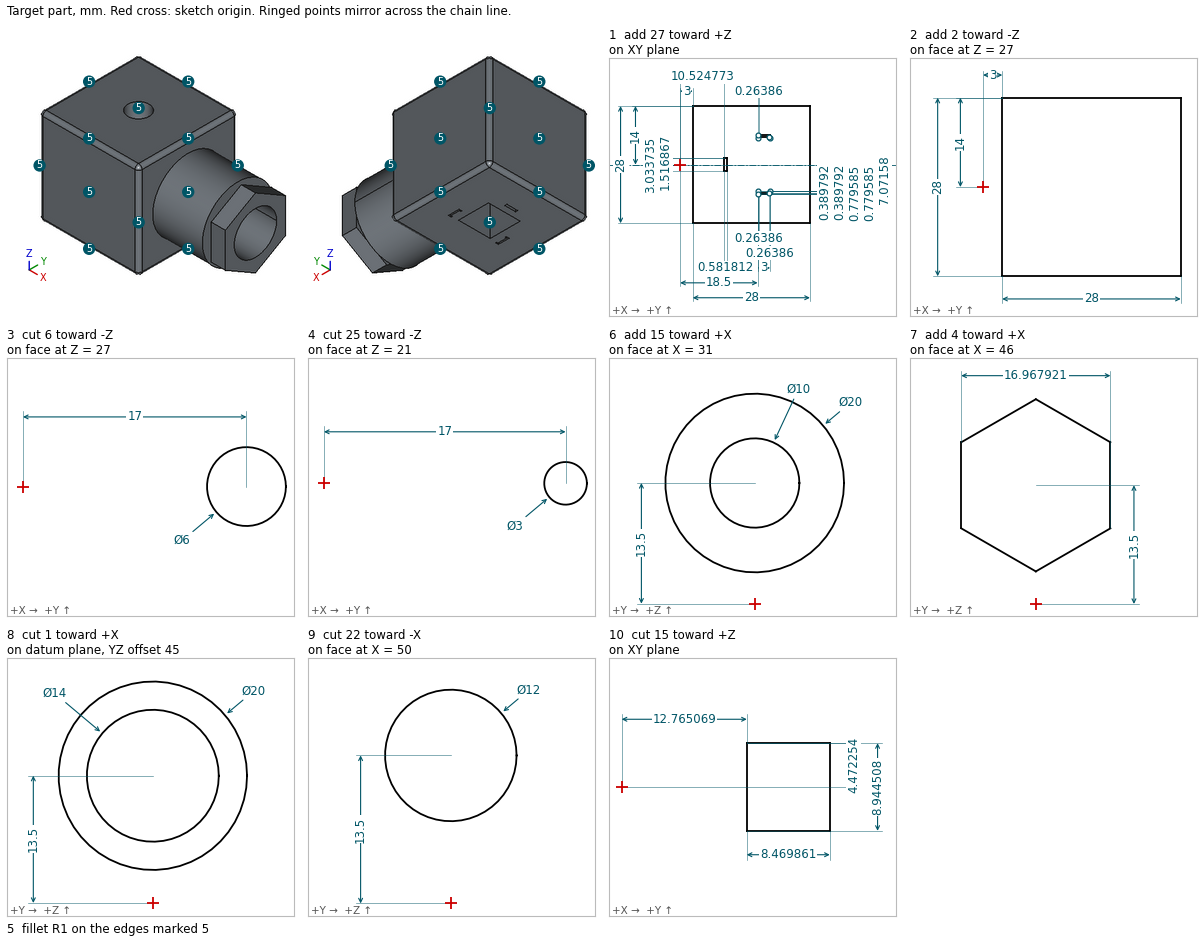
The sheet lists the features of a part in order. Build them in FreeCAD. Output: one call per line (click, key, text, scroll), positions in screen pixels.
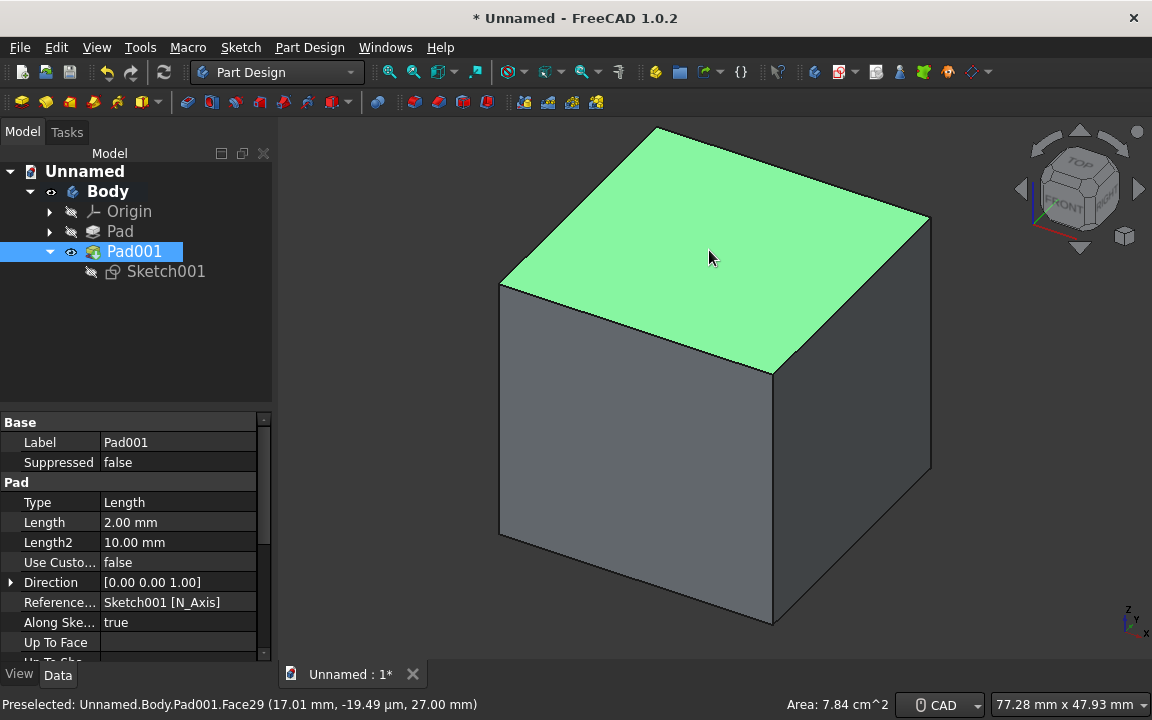
click(840, 72)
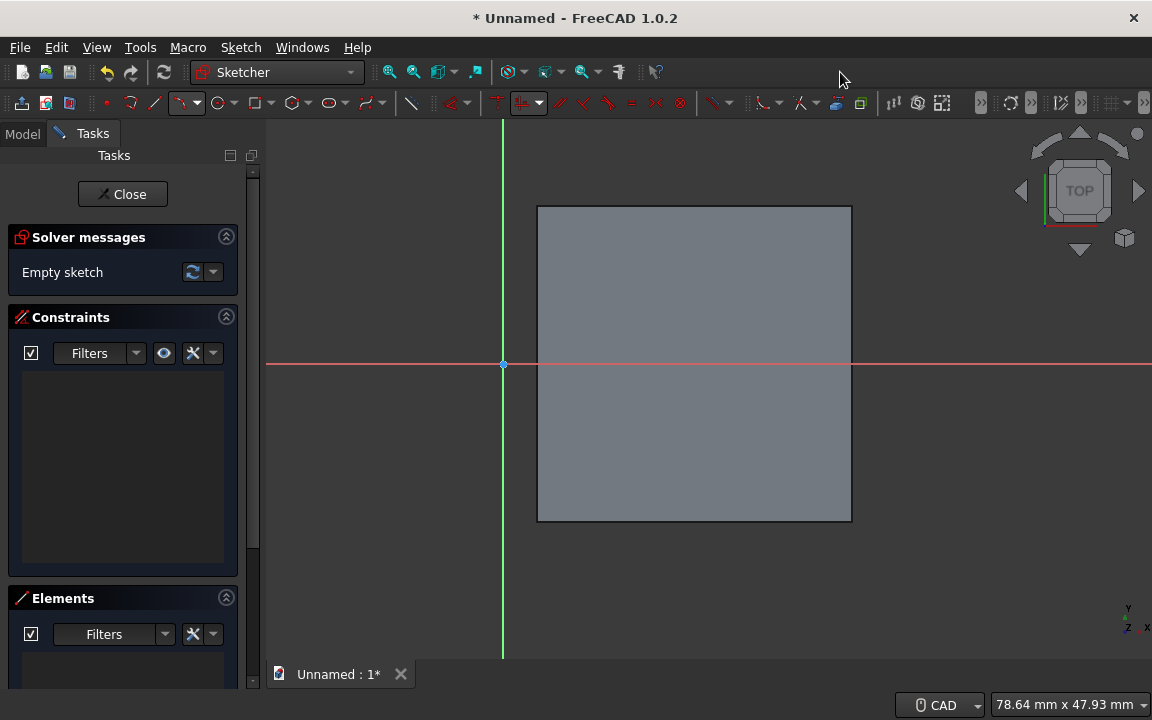
scroll(708, 358, up, 8)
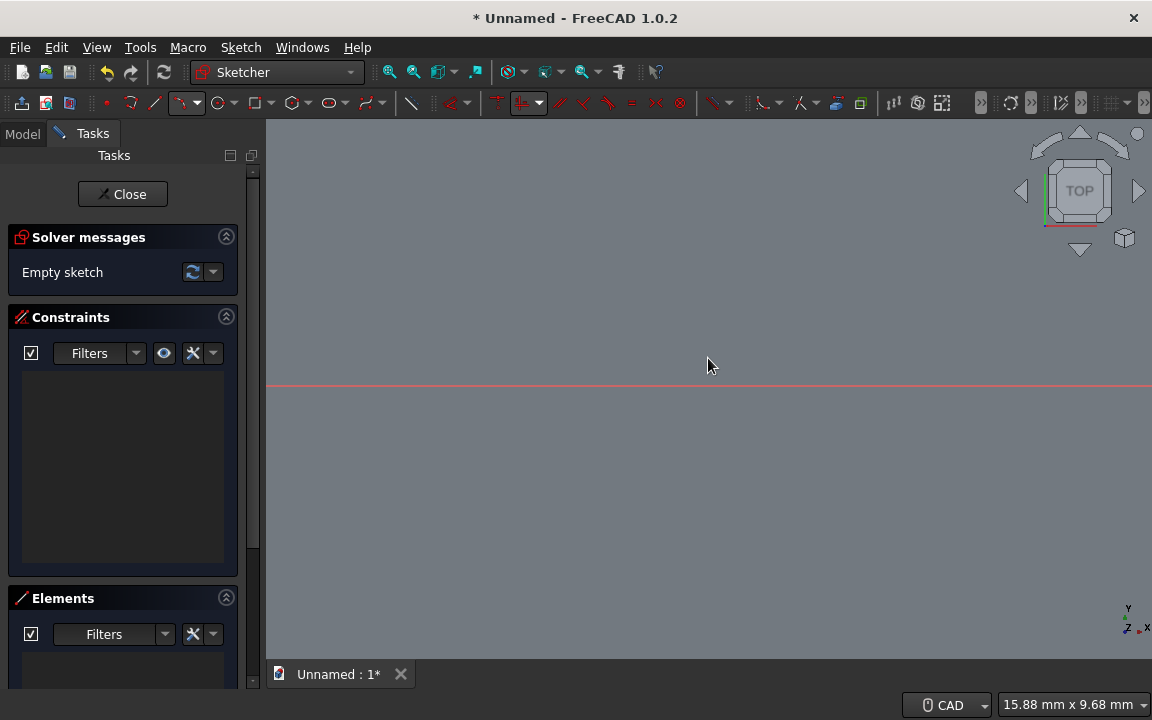
click(218, 104)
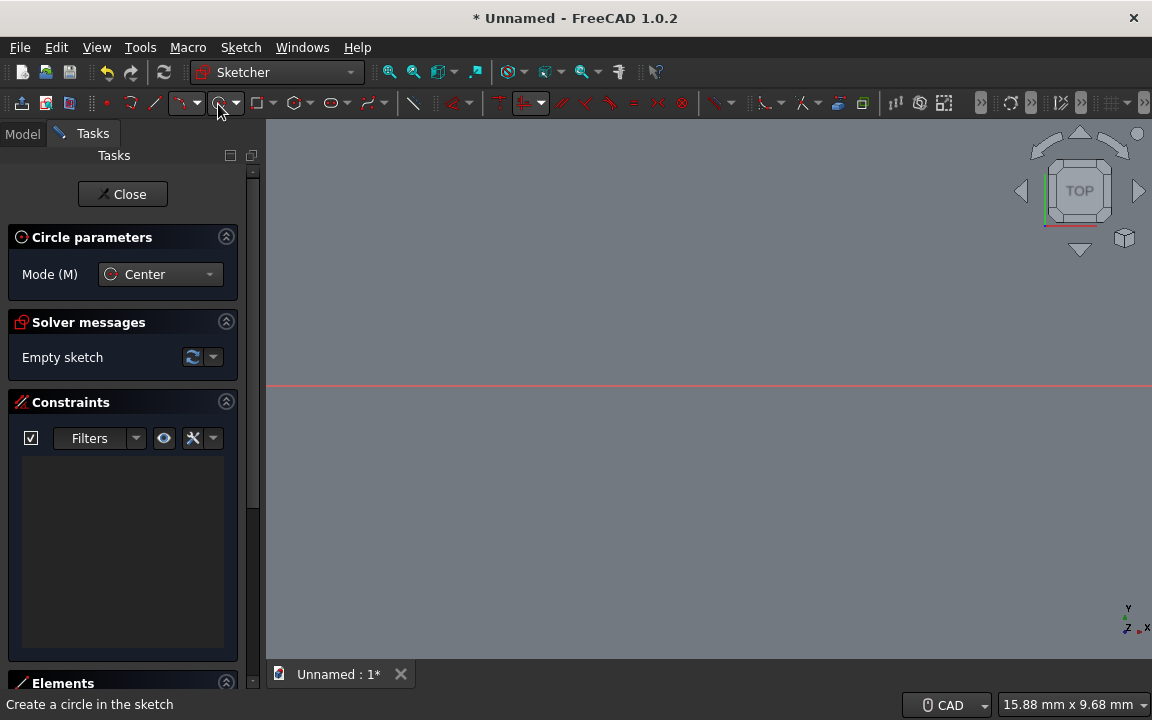
click(640, 386)
click(758, 268)
key(Escape)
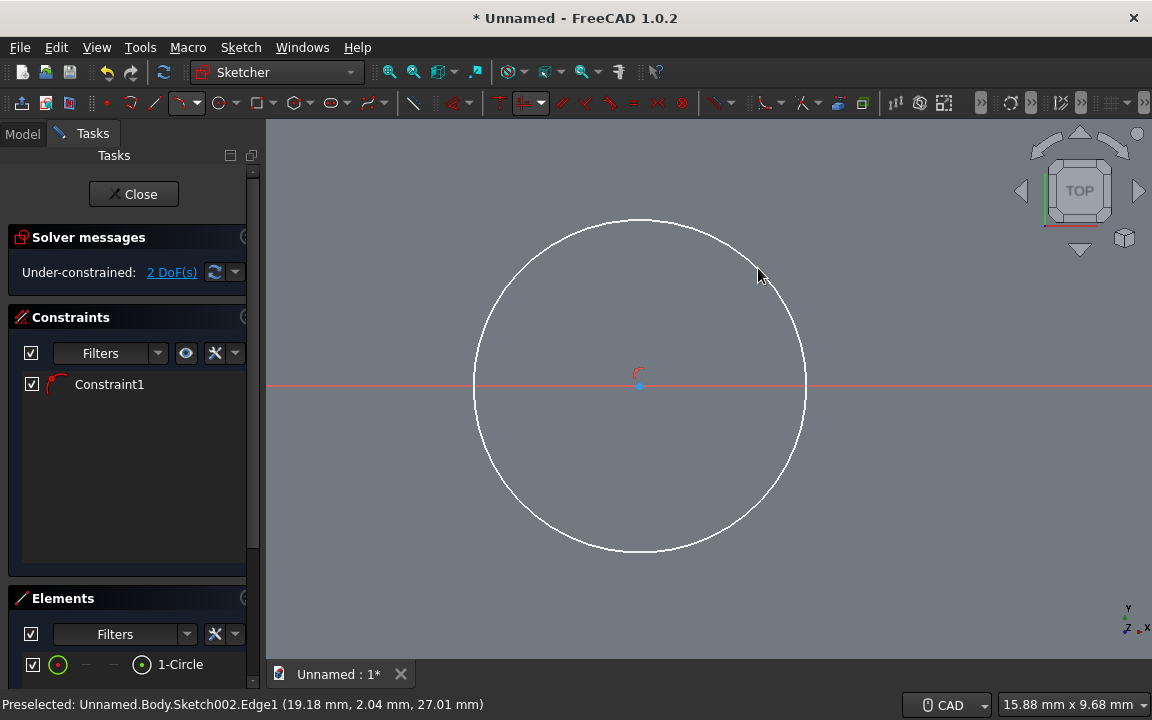
click(452, 104)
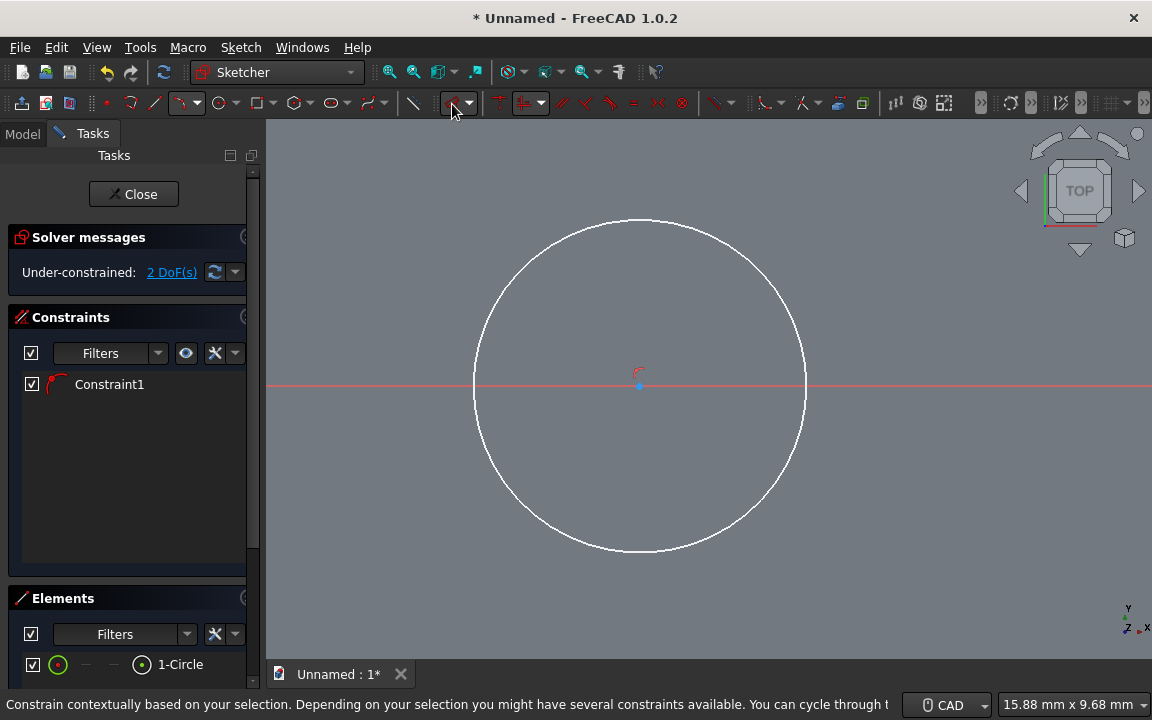
click(757, 268)
click(780, 245)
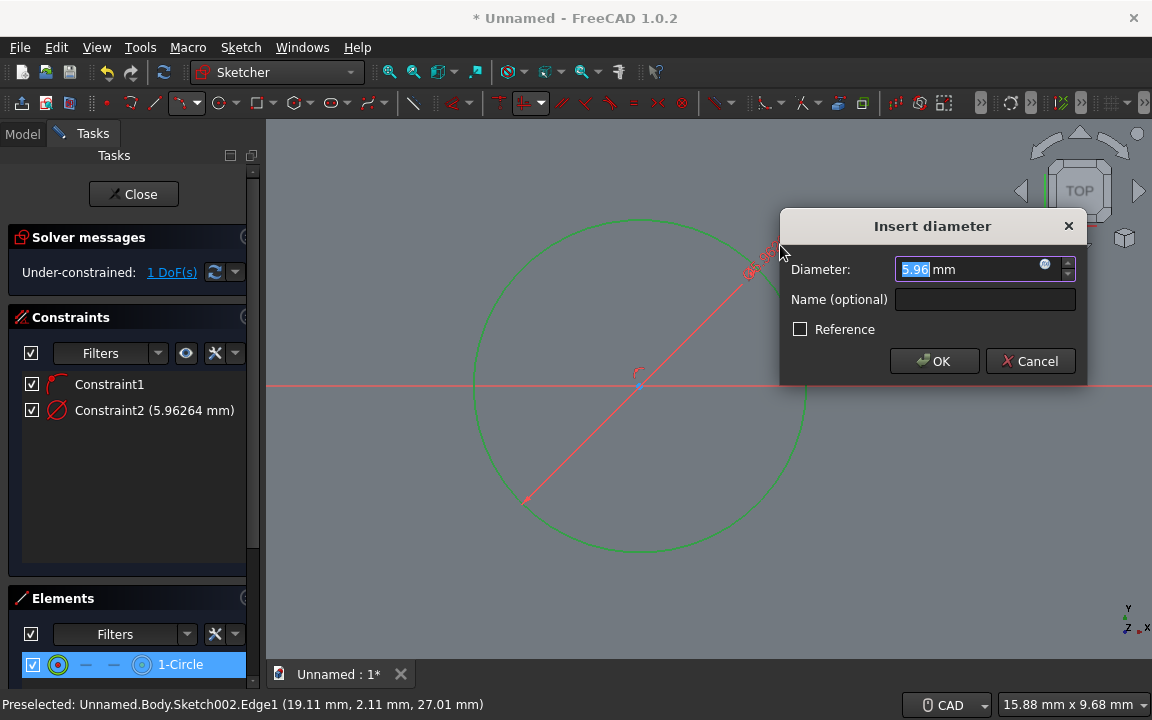
text(6)
key(Return)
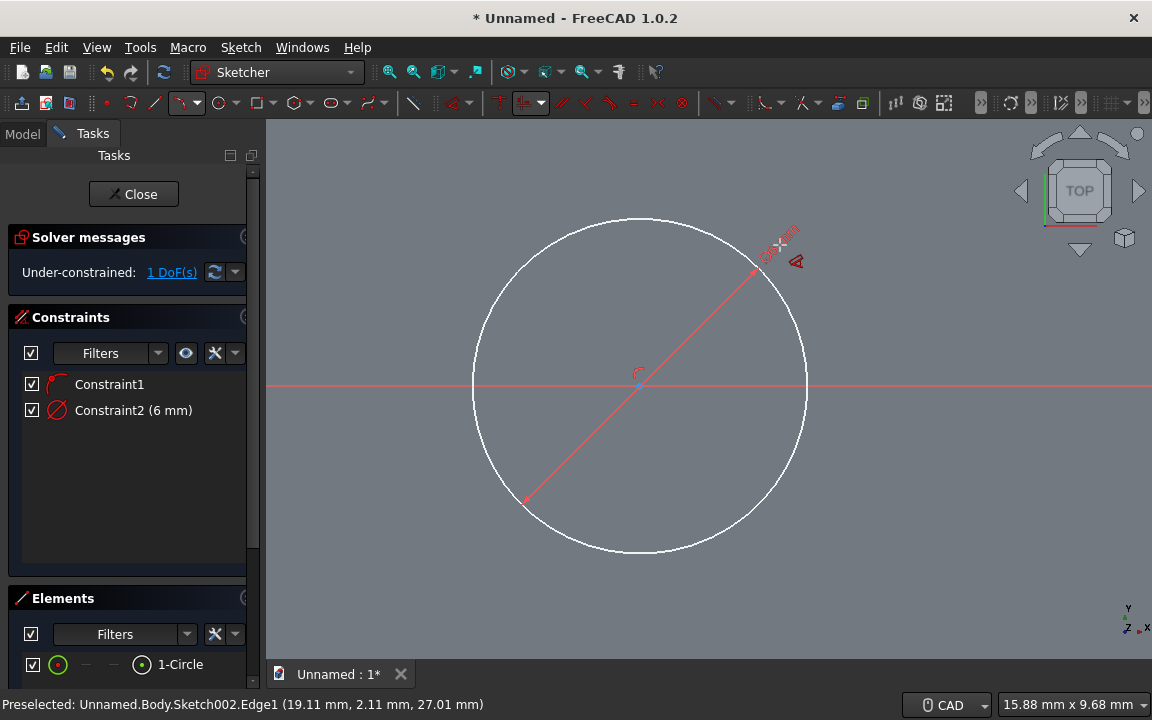
click(640, 386)
click(387, 420)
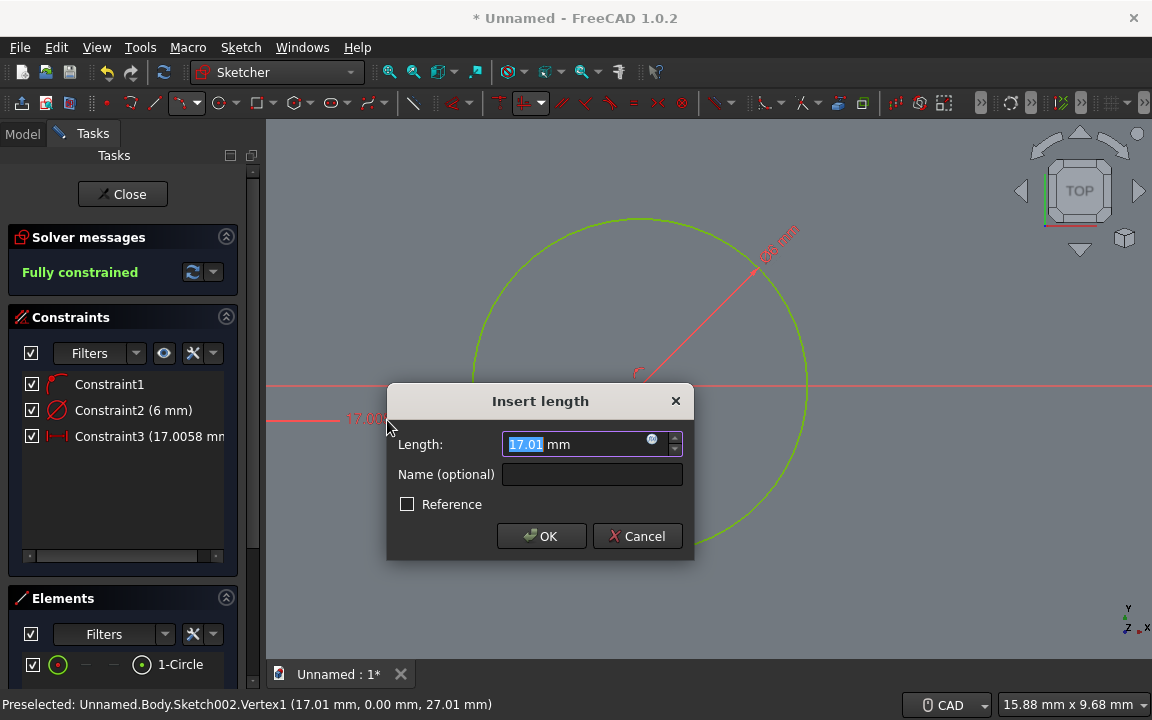
text(17)
key(Return)
key(Escape)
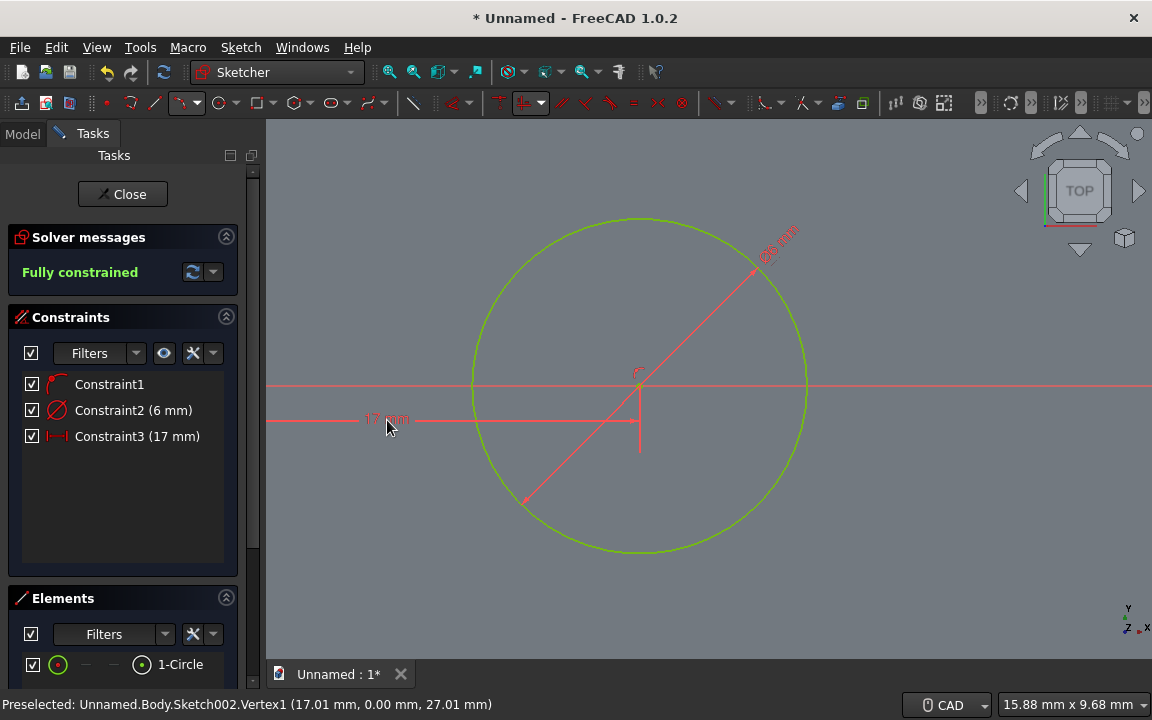
click(123, 194)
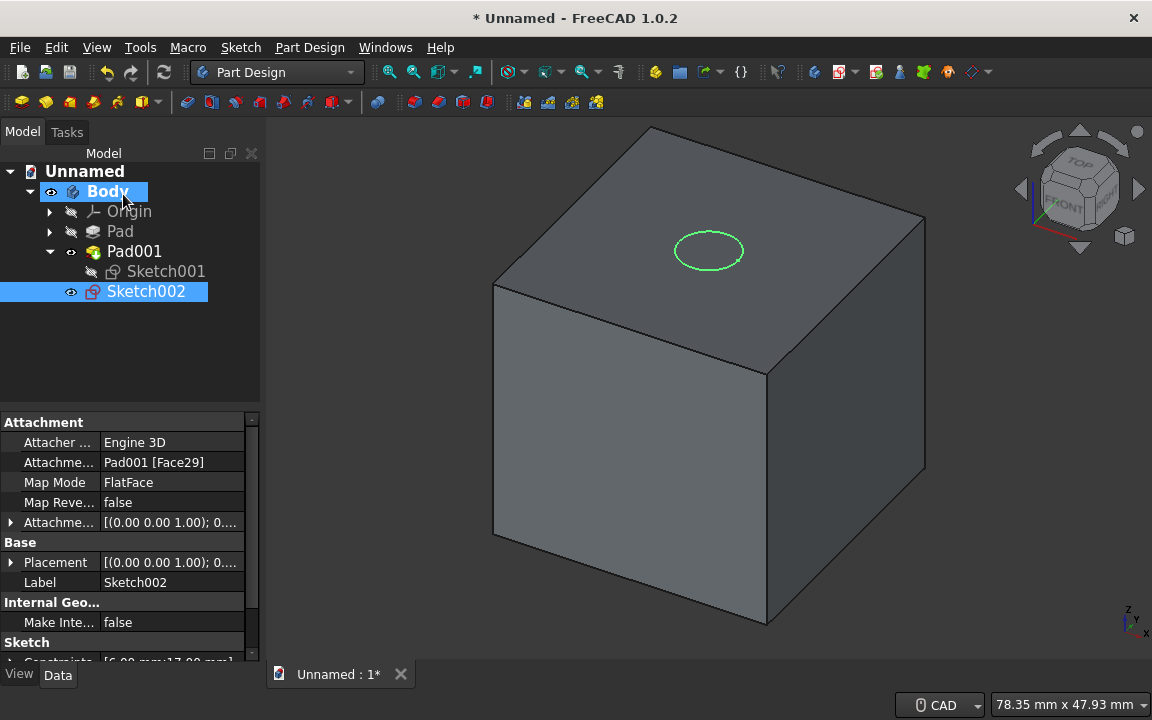
click(188, 102)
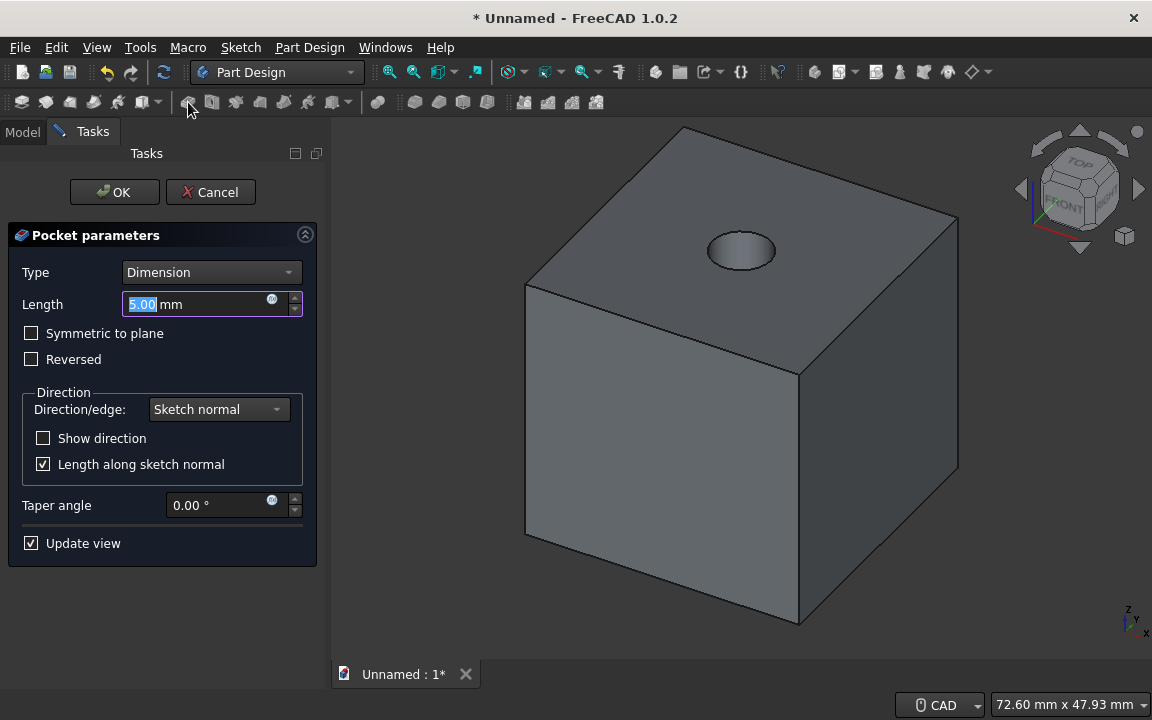
text(6)
key(Tab)